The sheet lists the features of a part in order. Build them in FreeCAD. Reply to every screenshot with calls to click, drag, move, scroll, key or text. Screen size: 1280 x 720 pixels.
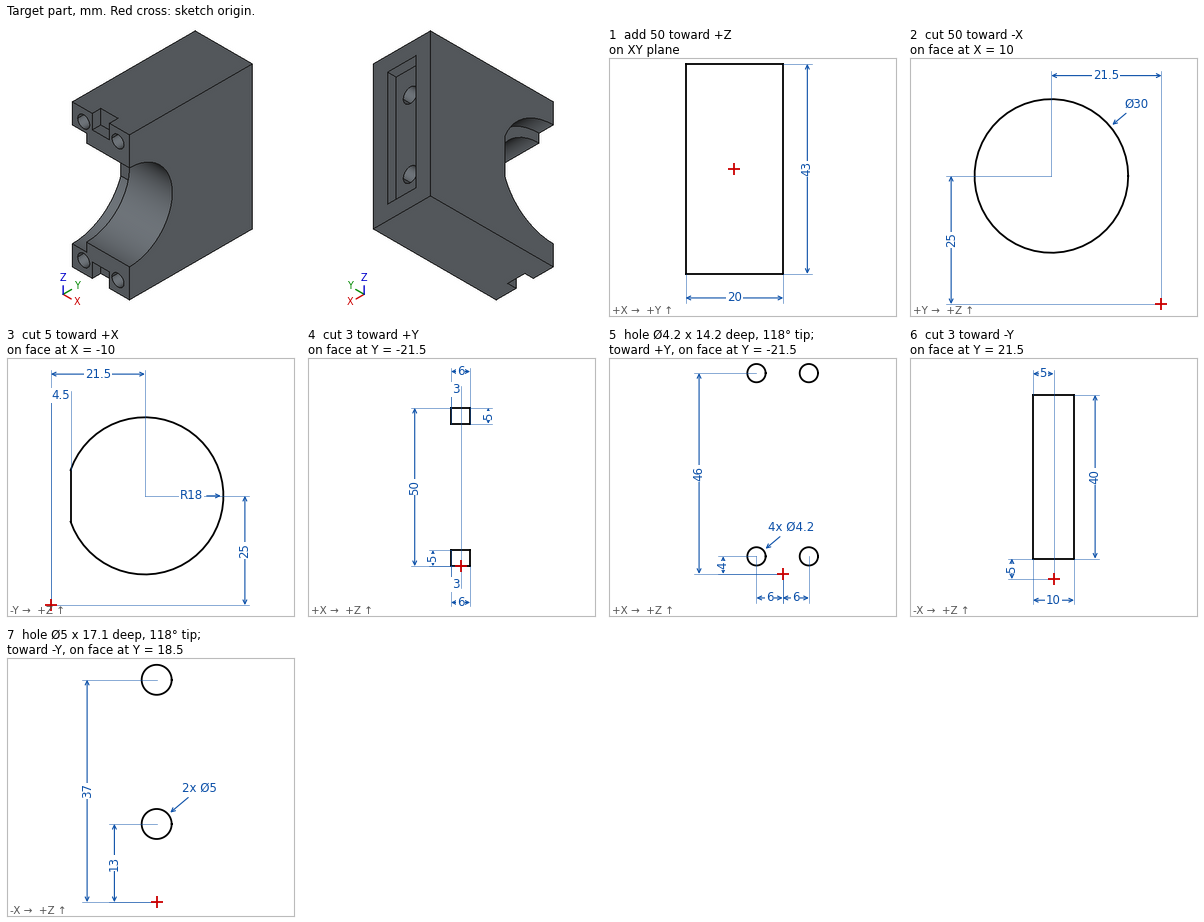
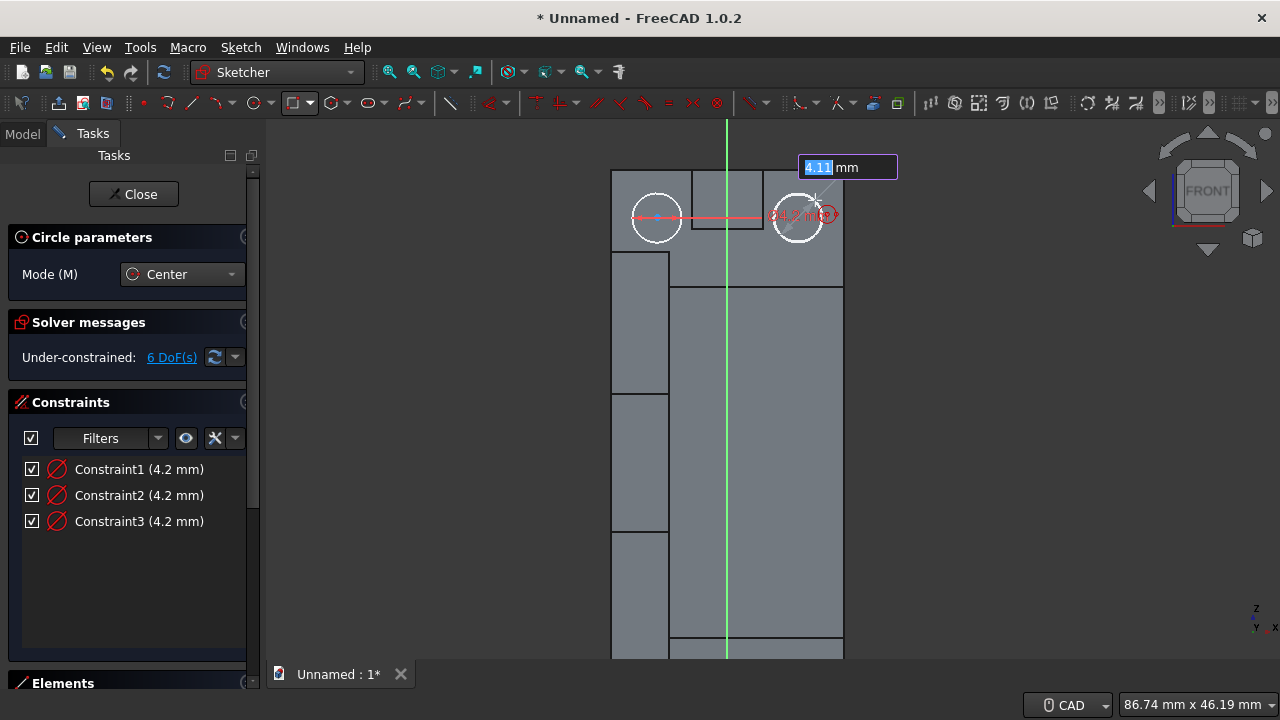
text(4.2)
key(Return)
key(Escape)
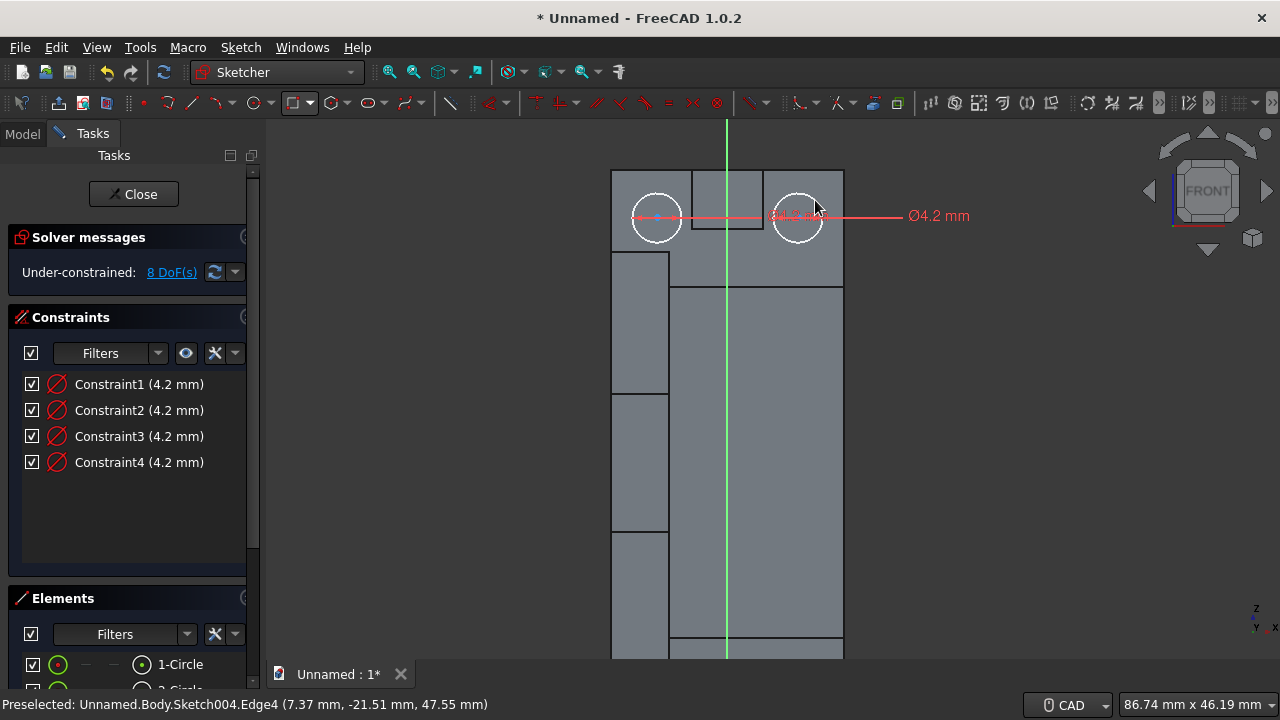
scroll(658, 217, down, 2)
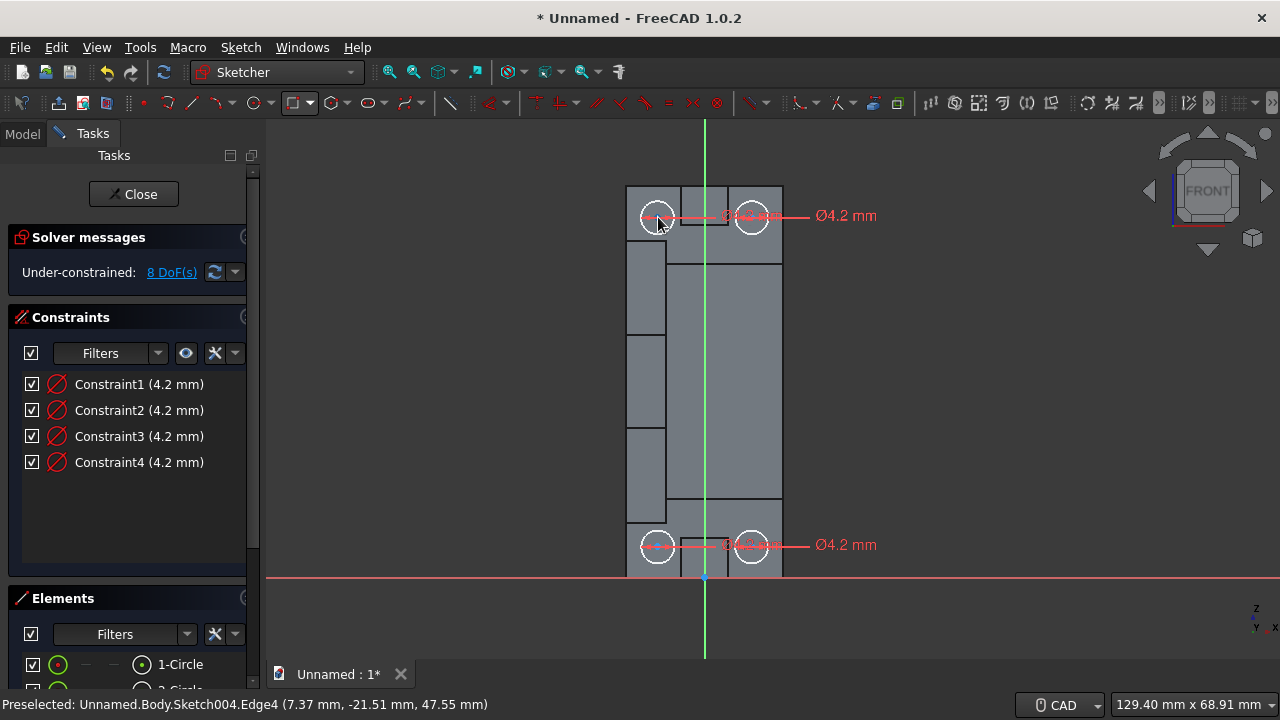
click(658, 547)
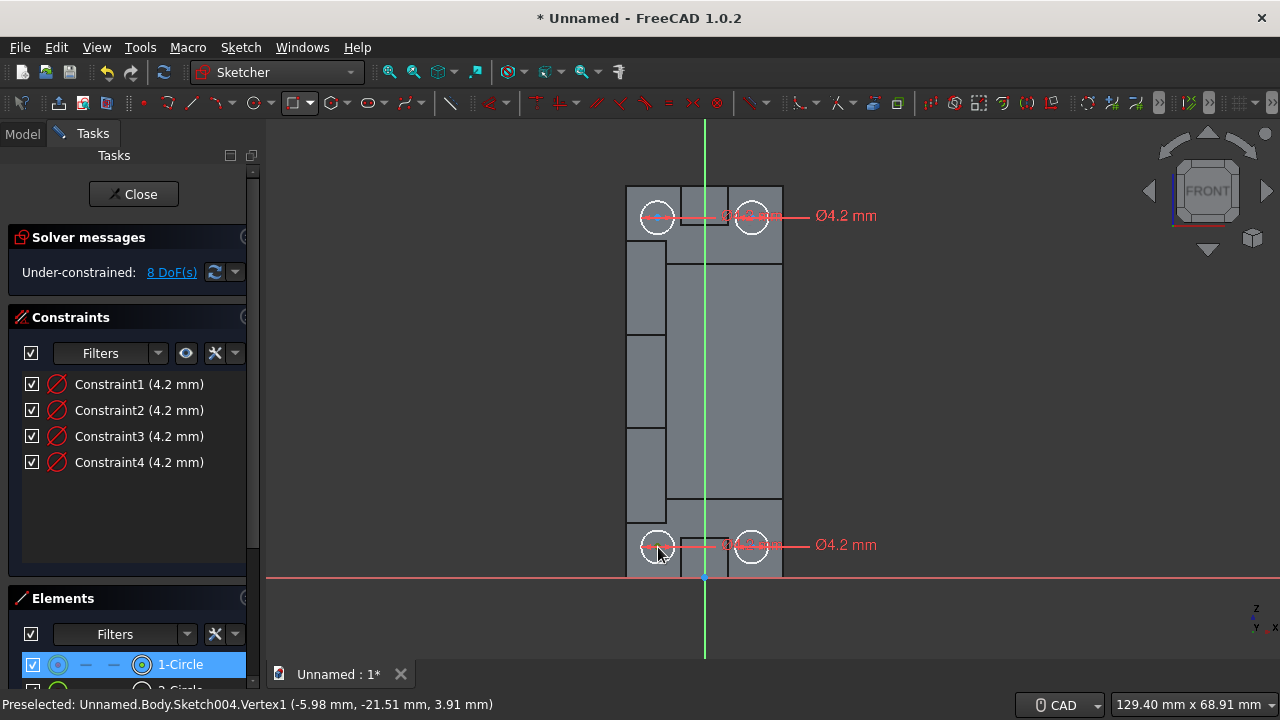
click(752, 547)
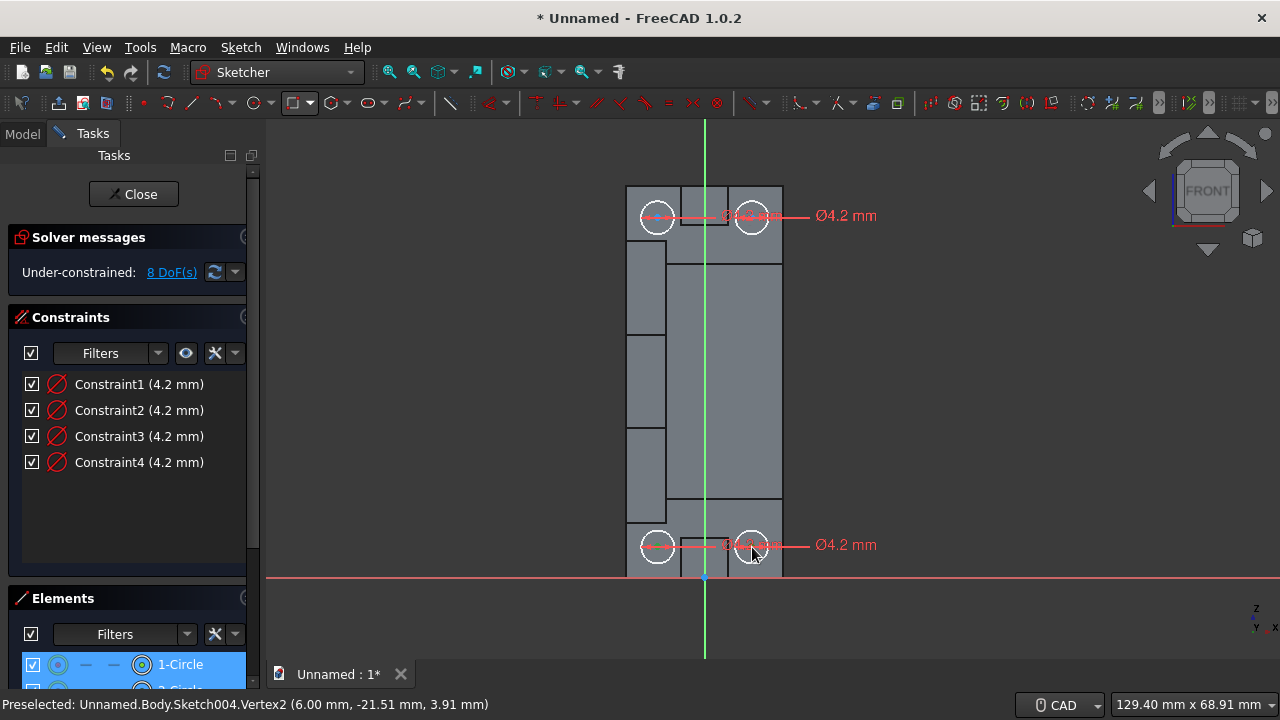
click(578, 104)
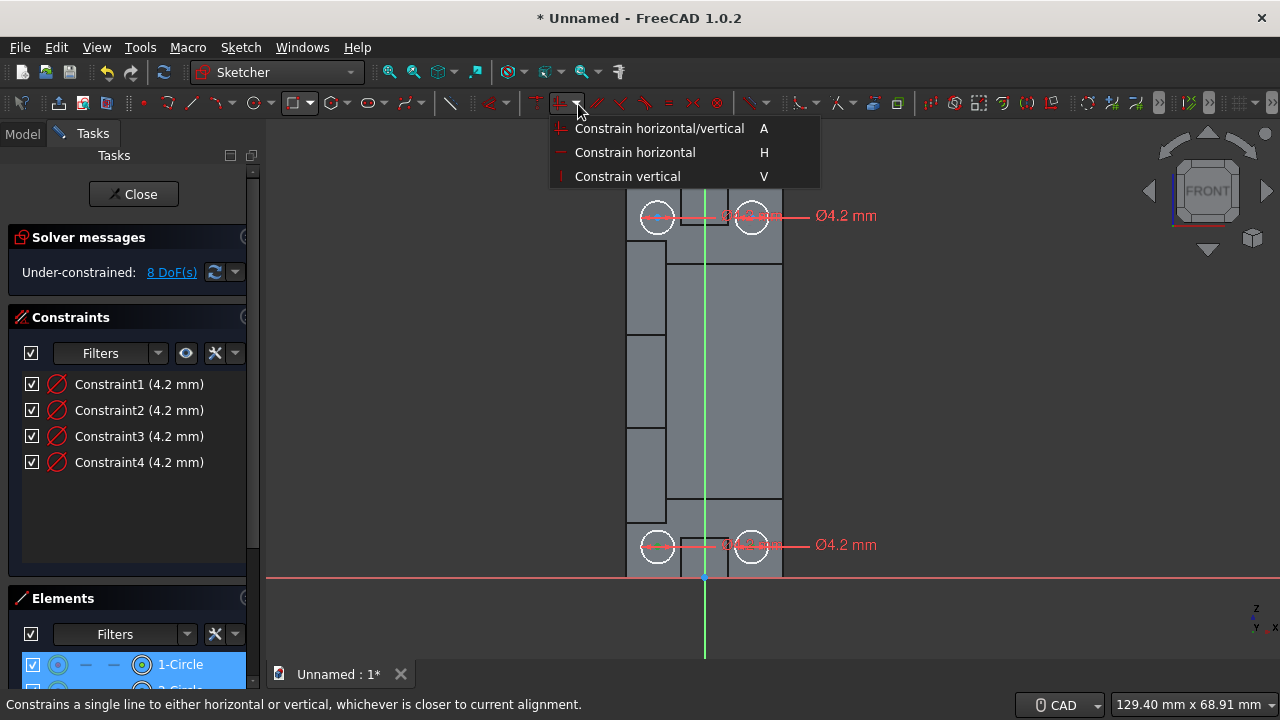
click(685, 152)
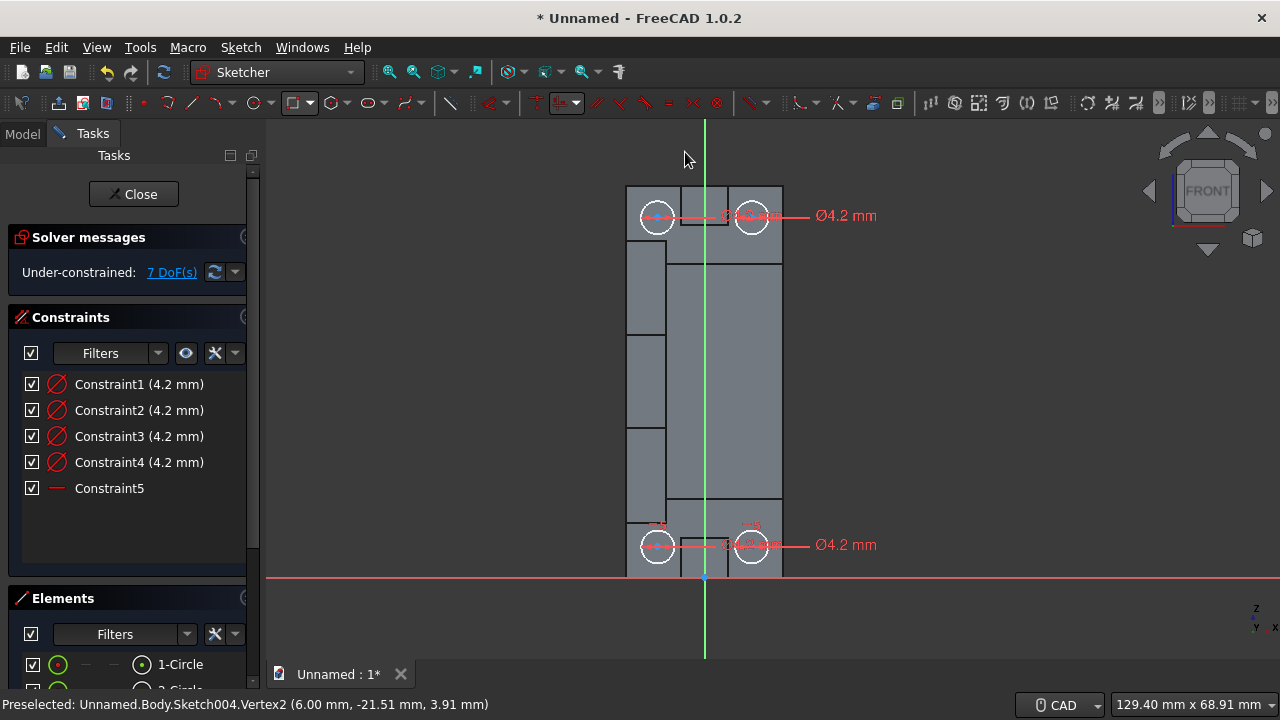
click(658, 547)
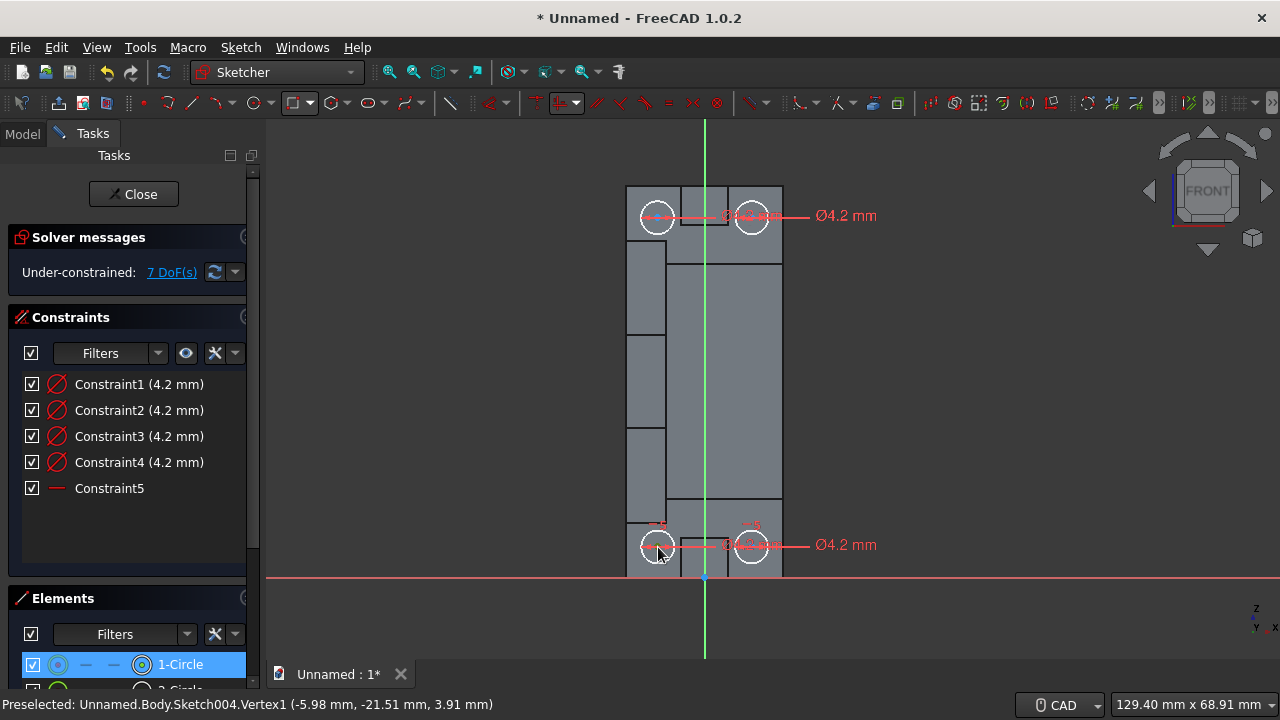
click(657, 218)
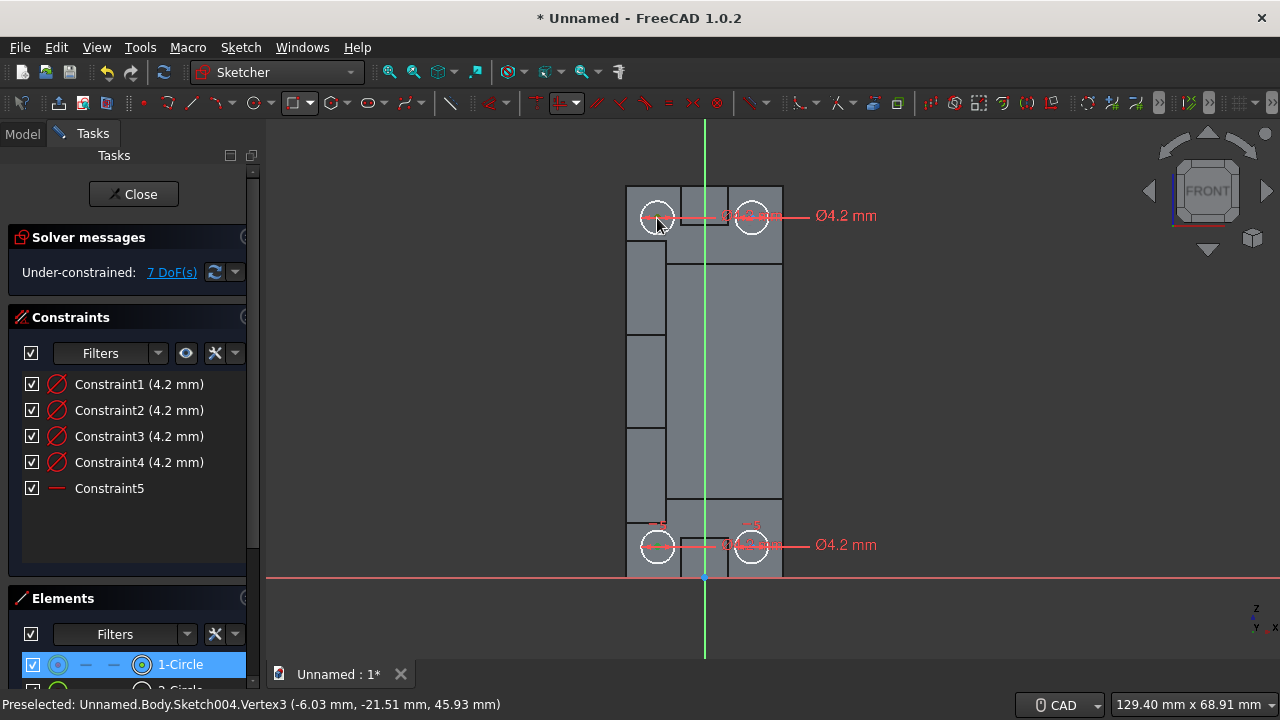
key(v)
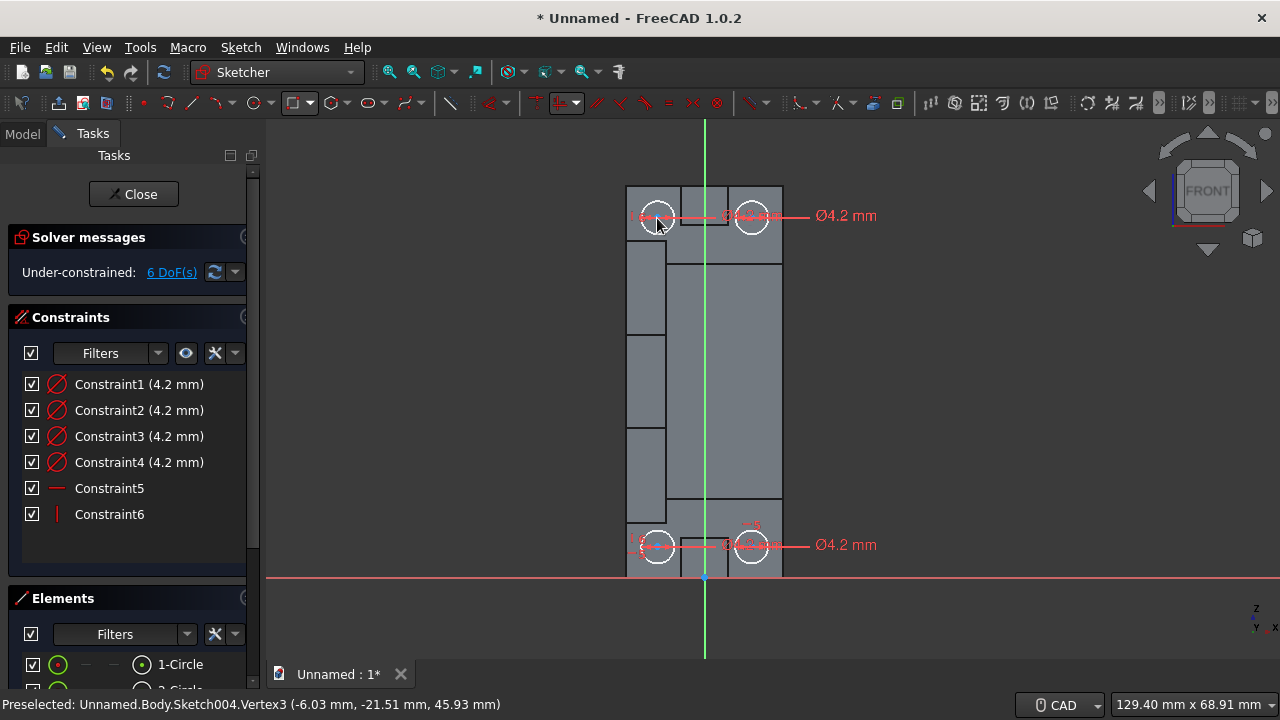
click(752, 547)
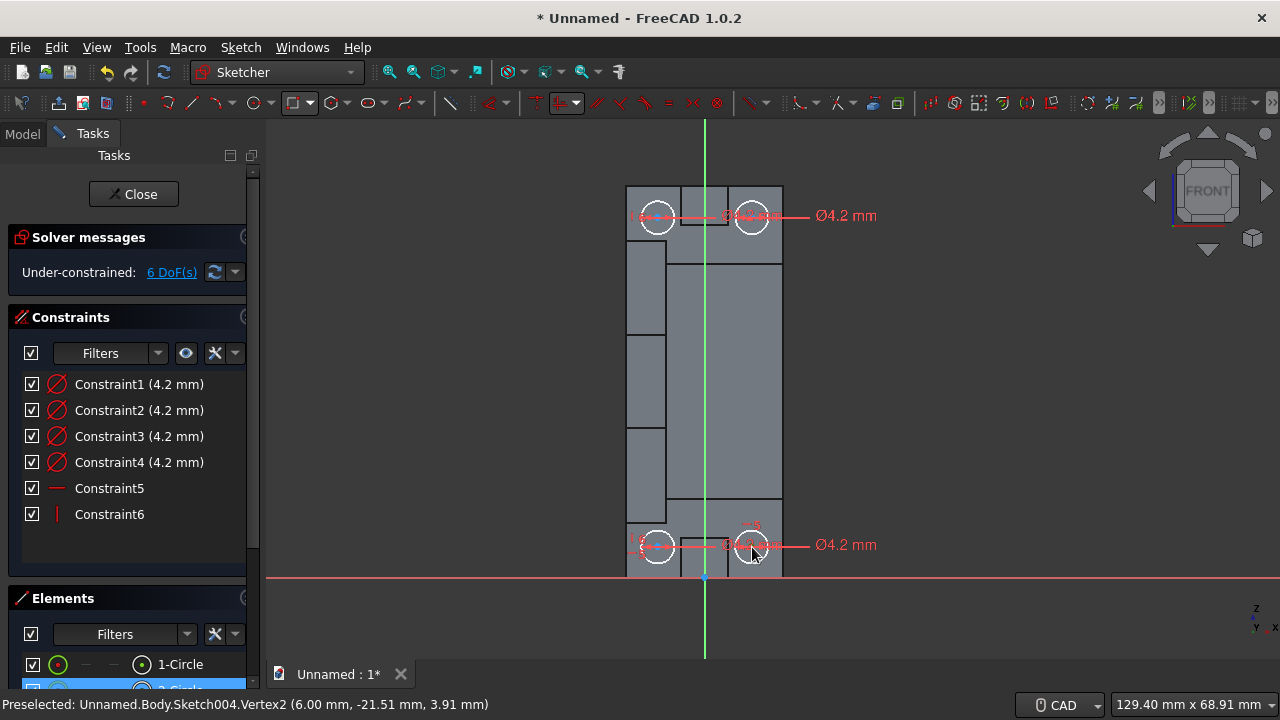
click(752, 218)